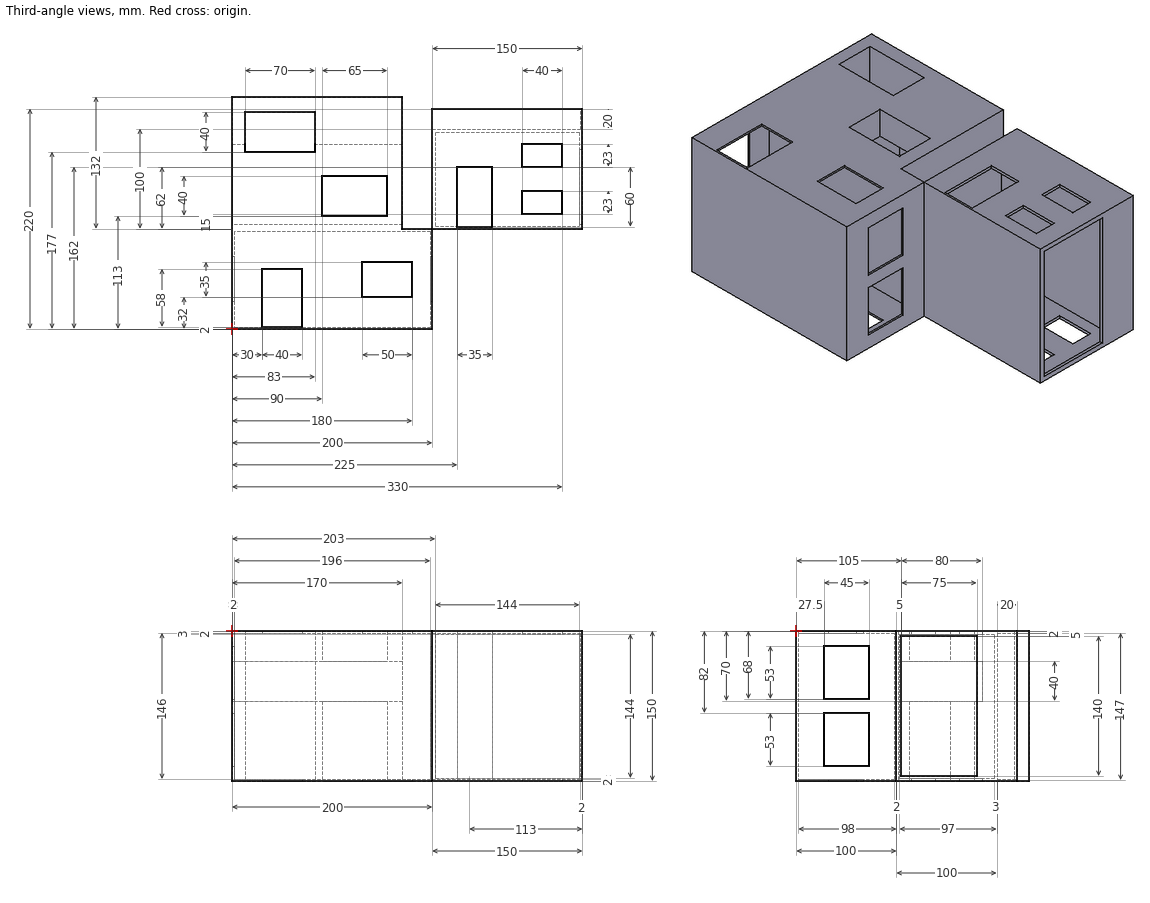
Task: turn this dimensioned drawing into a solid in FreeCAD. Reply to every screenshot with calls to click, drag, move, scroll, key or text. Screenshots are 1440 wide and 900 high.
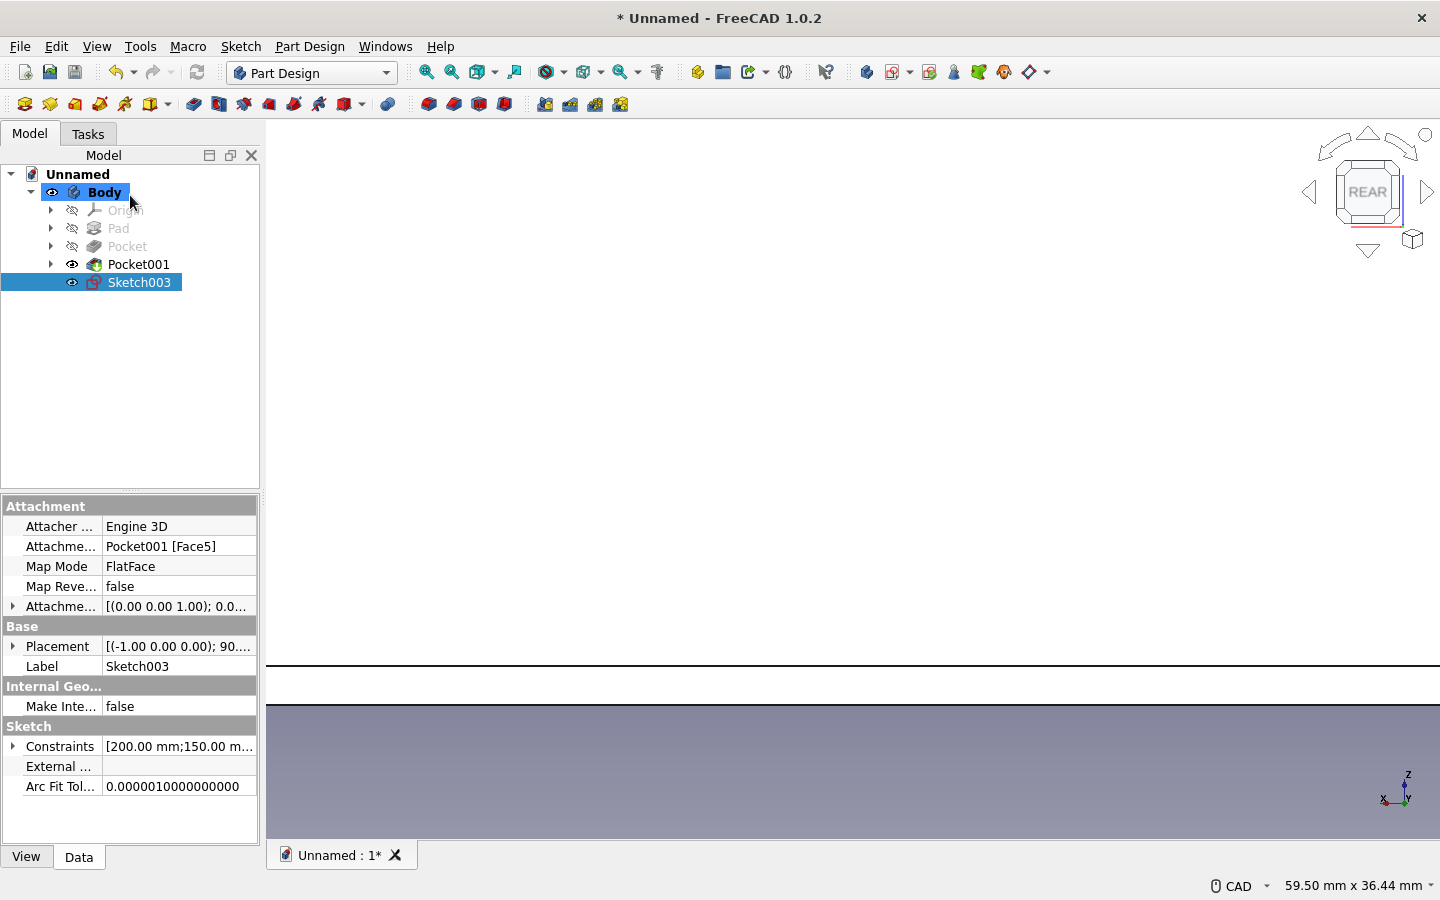
click(25, 104)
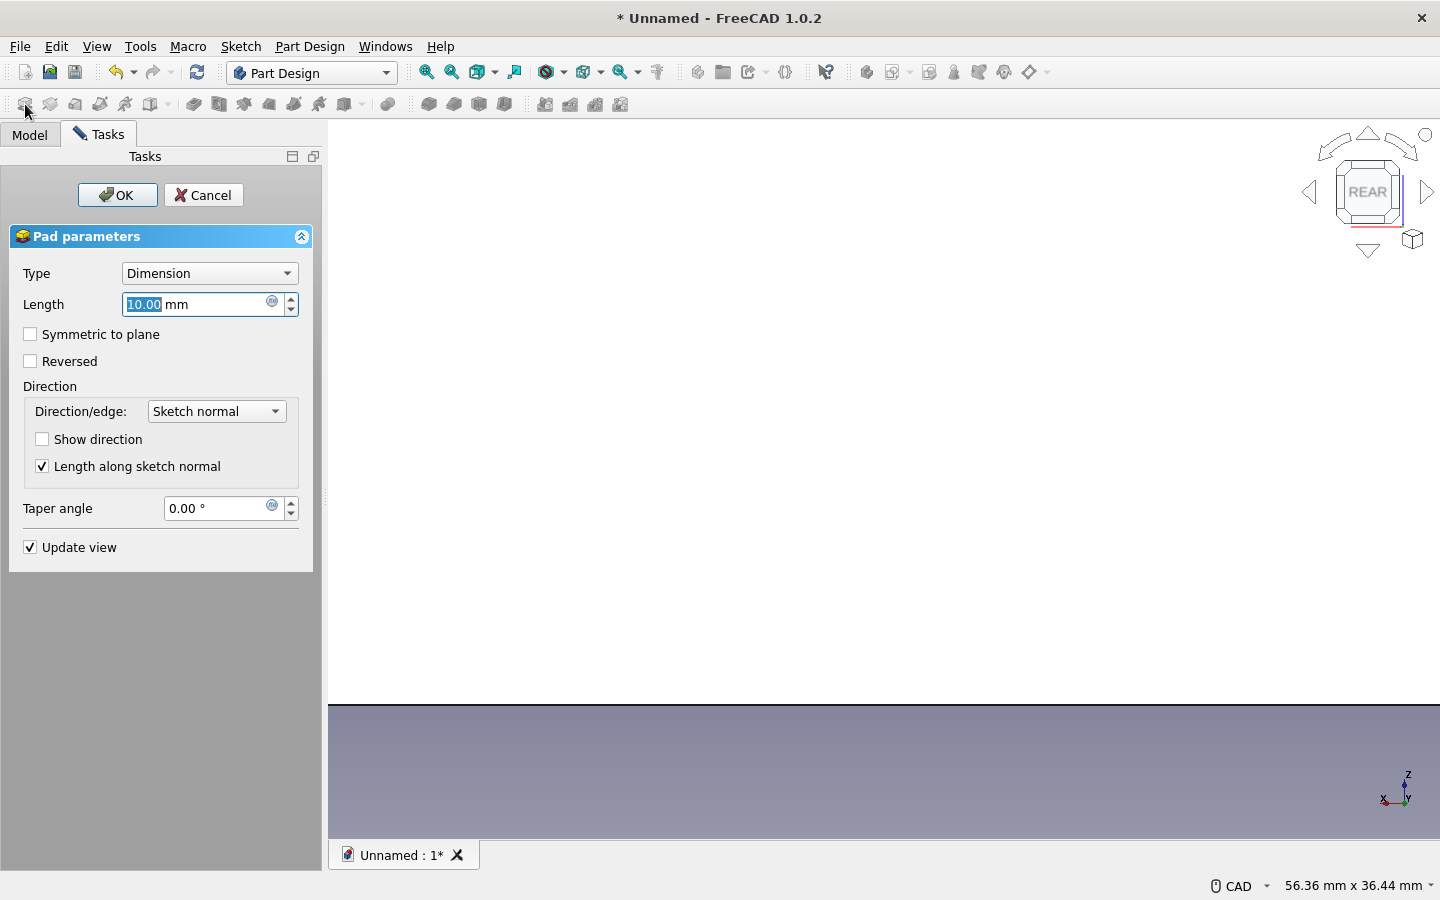
text(2)
key(Tab)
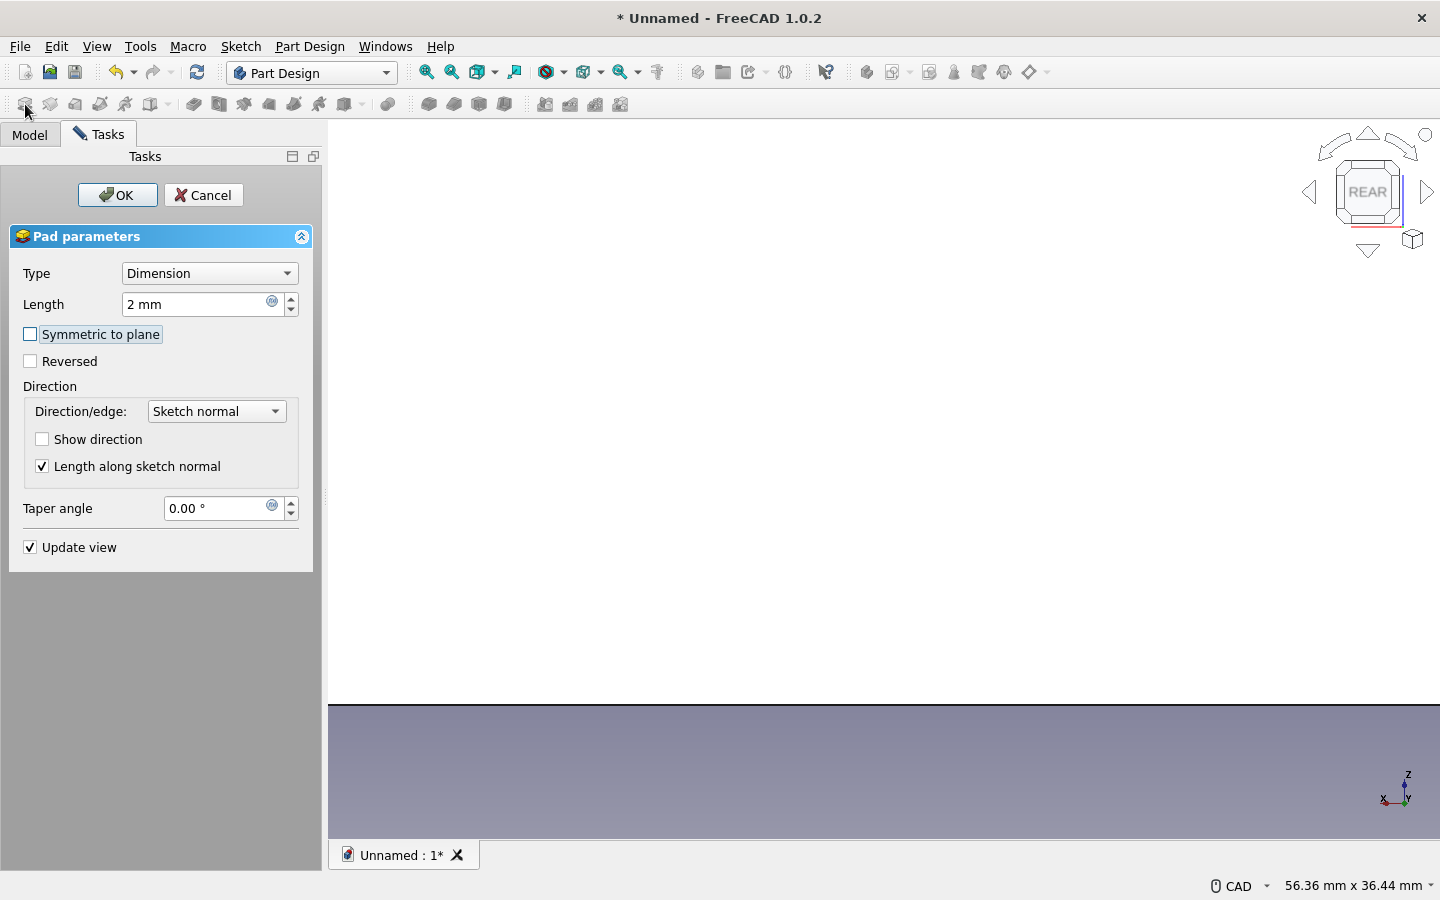
click(31, 361)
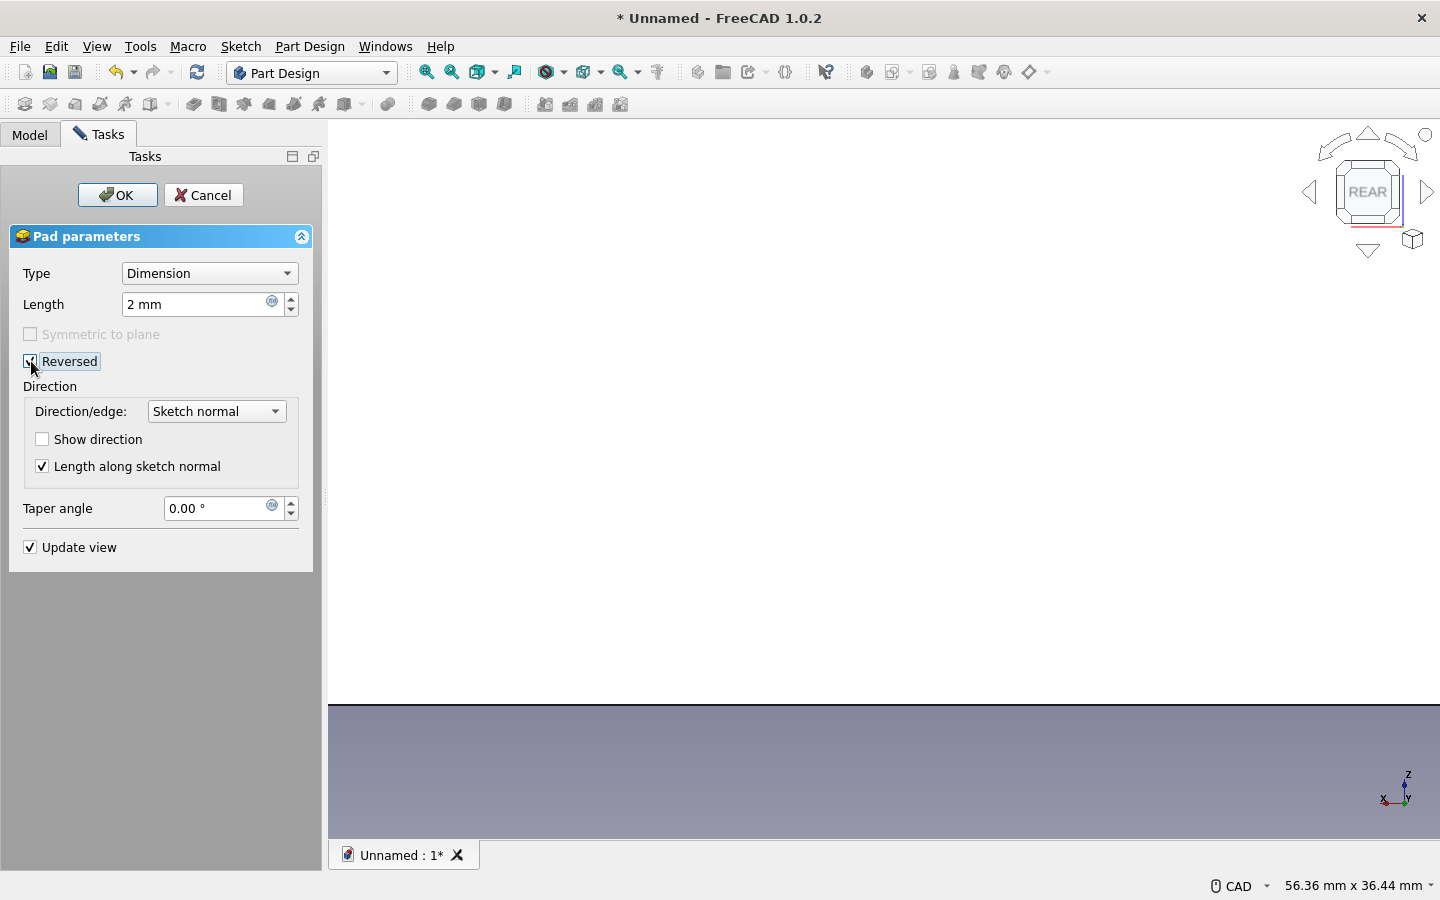
click(118, 195)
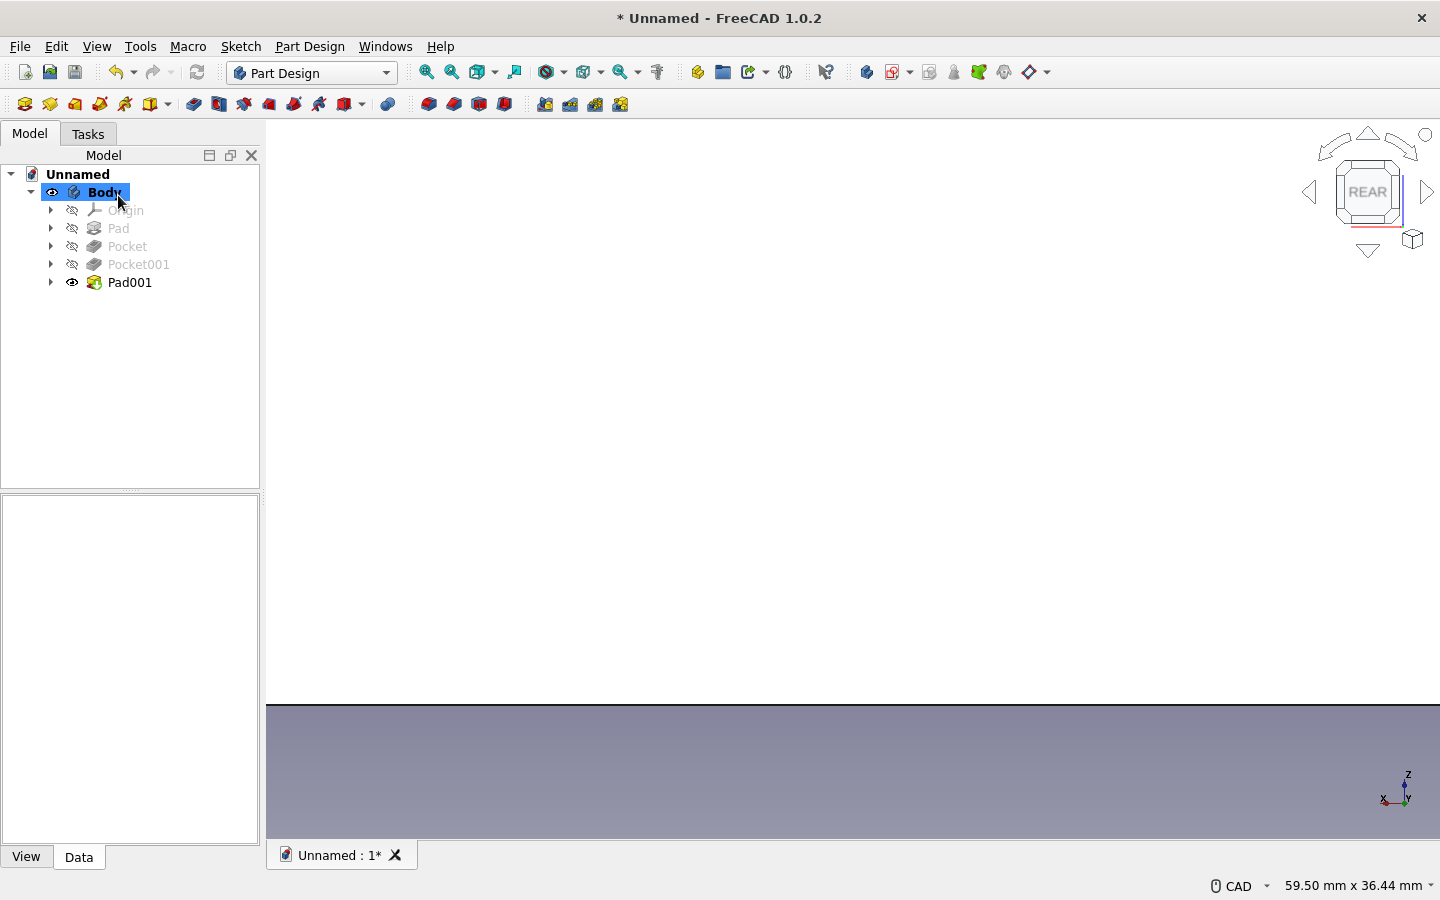
click(427, 72)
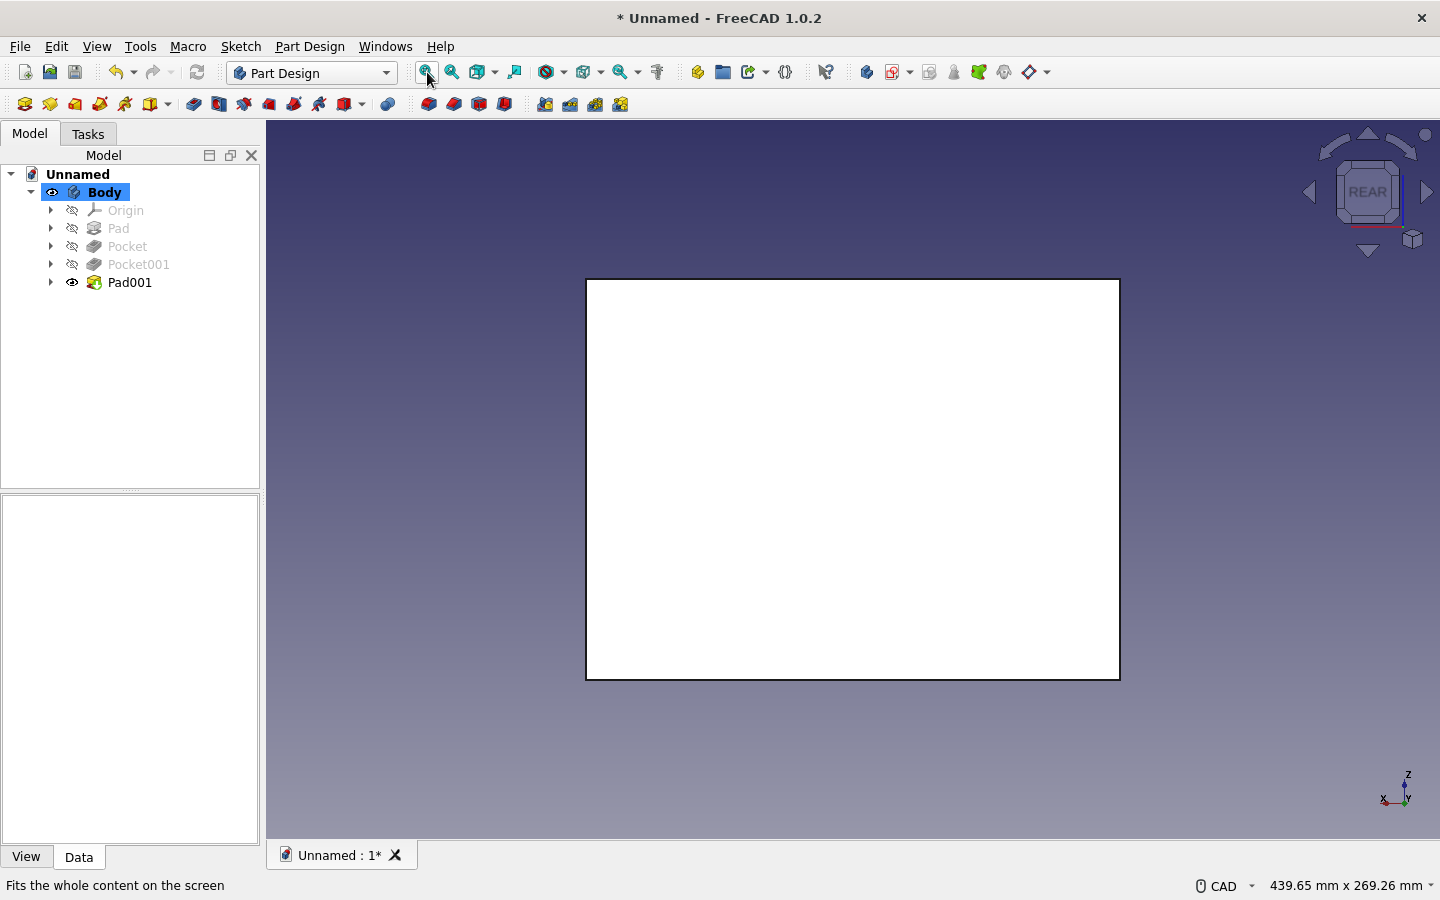
key(0)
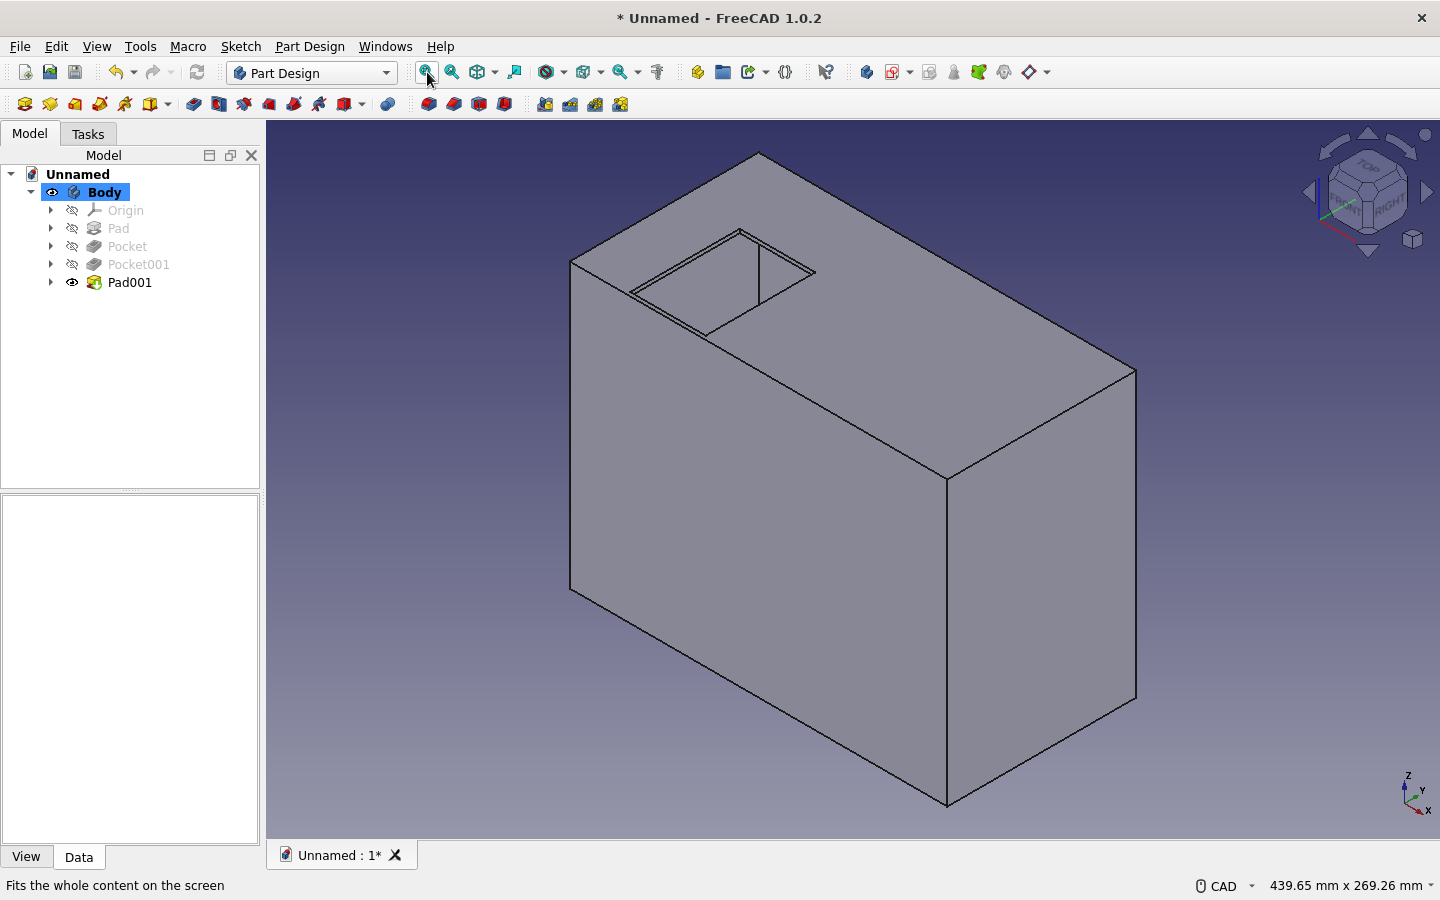
click(907, 346)